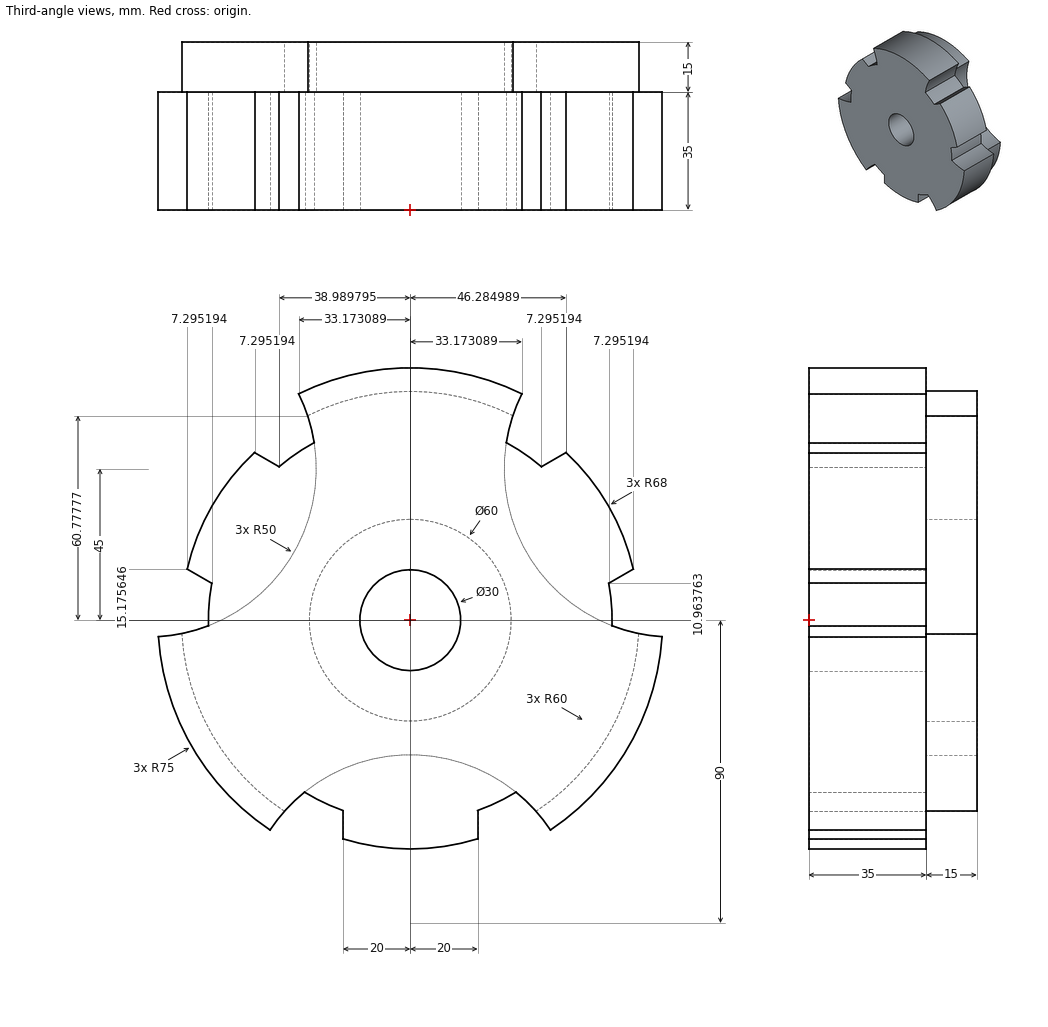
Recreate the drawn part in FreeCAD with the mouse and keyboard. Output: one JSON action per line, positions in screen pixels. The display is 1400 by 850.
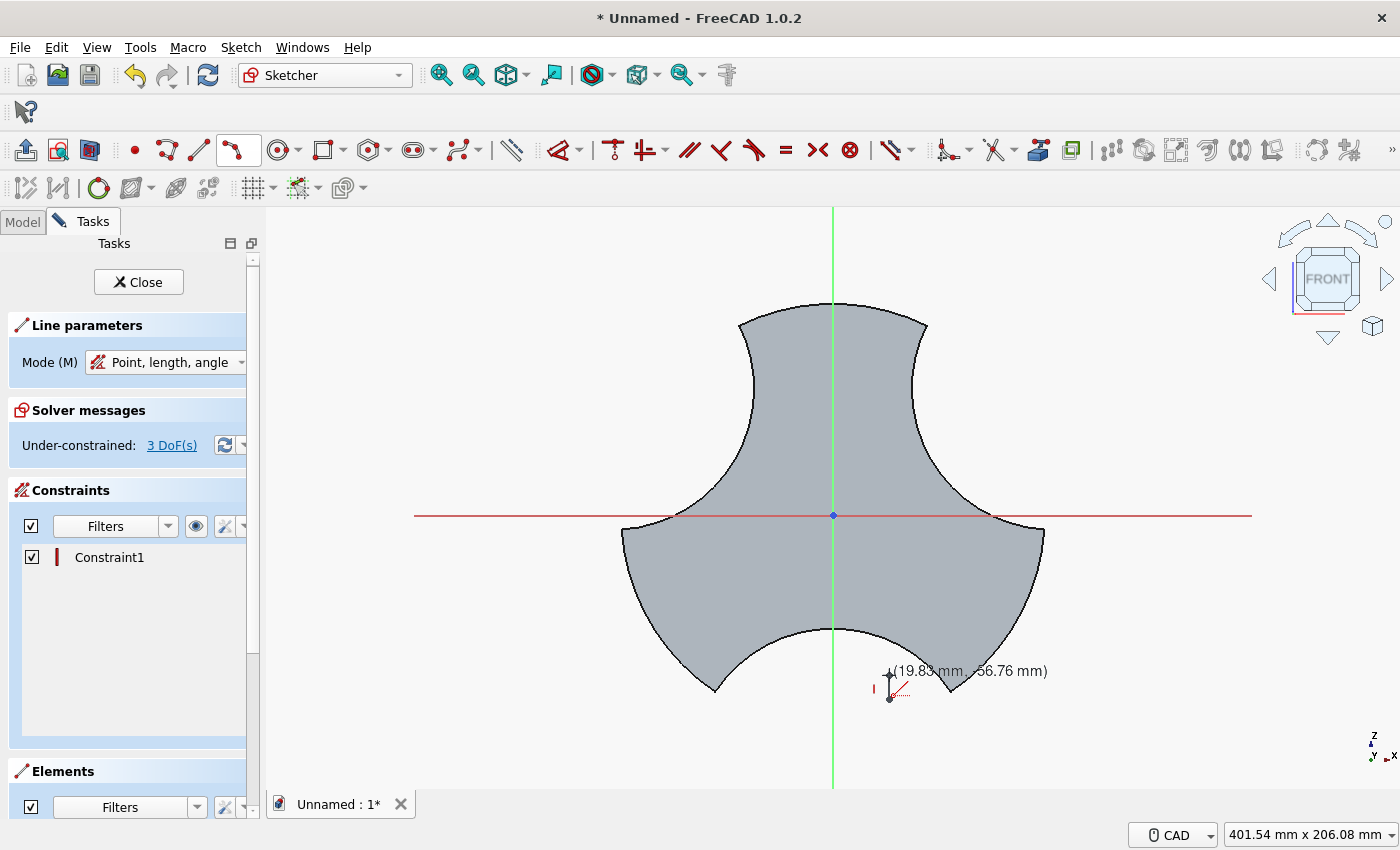
{"action": "left_click", "coordinate": [1000, 485]}
{"action": "left_click", "coordinate": [1020, 473]}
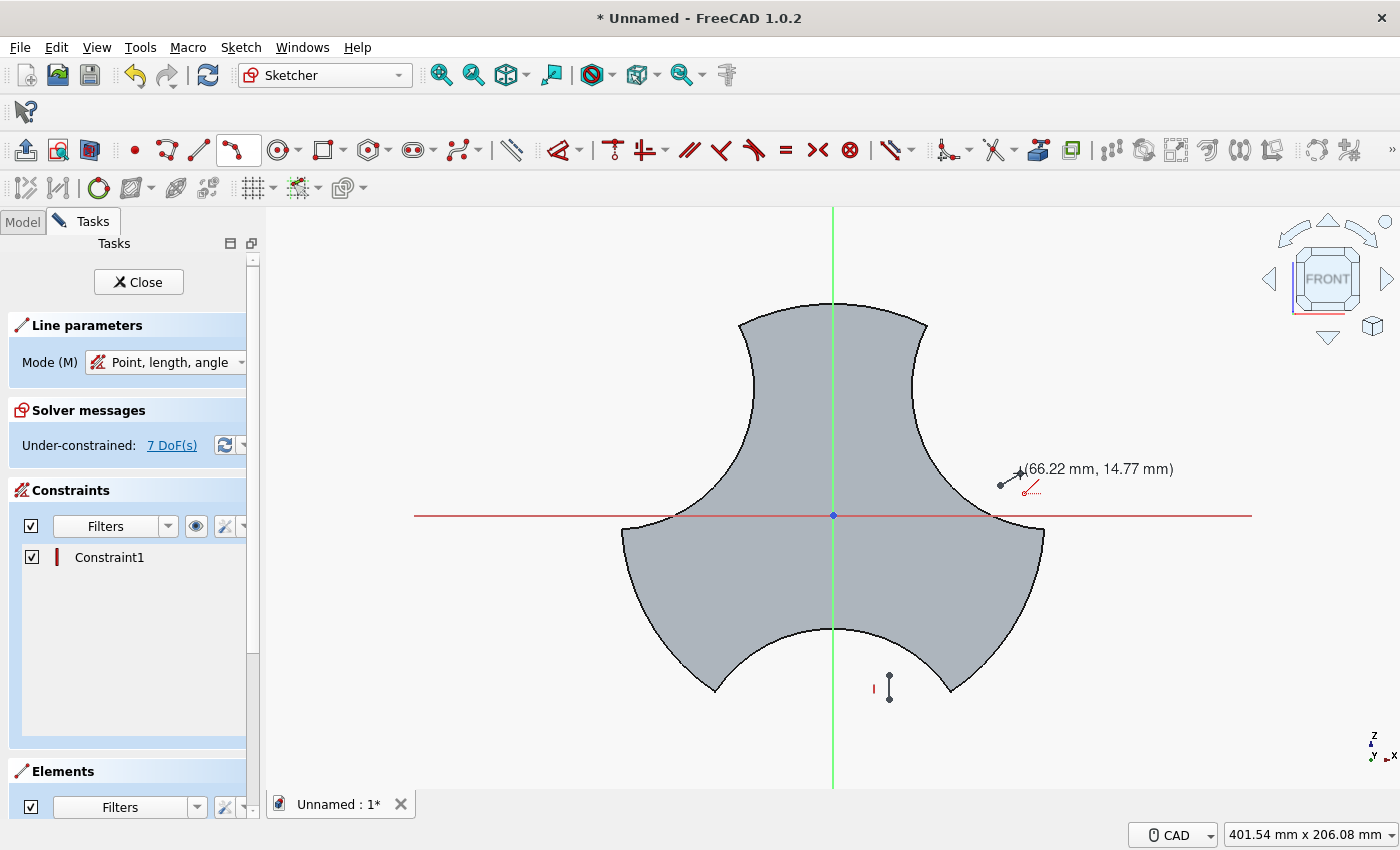
{"action": "left_click", "coordinate": [964, 375]}
{"action": "left_click", "coordinate": [943, 387]}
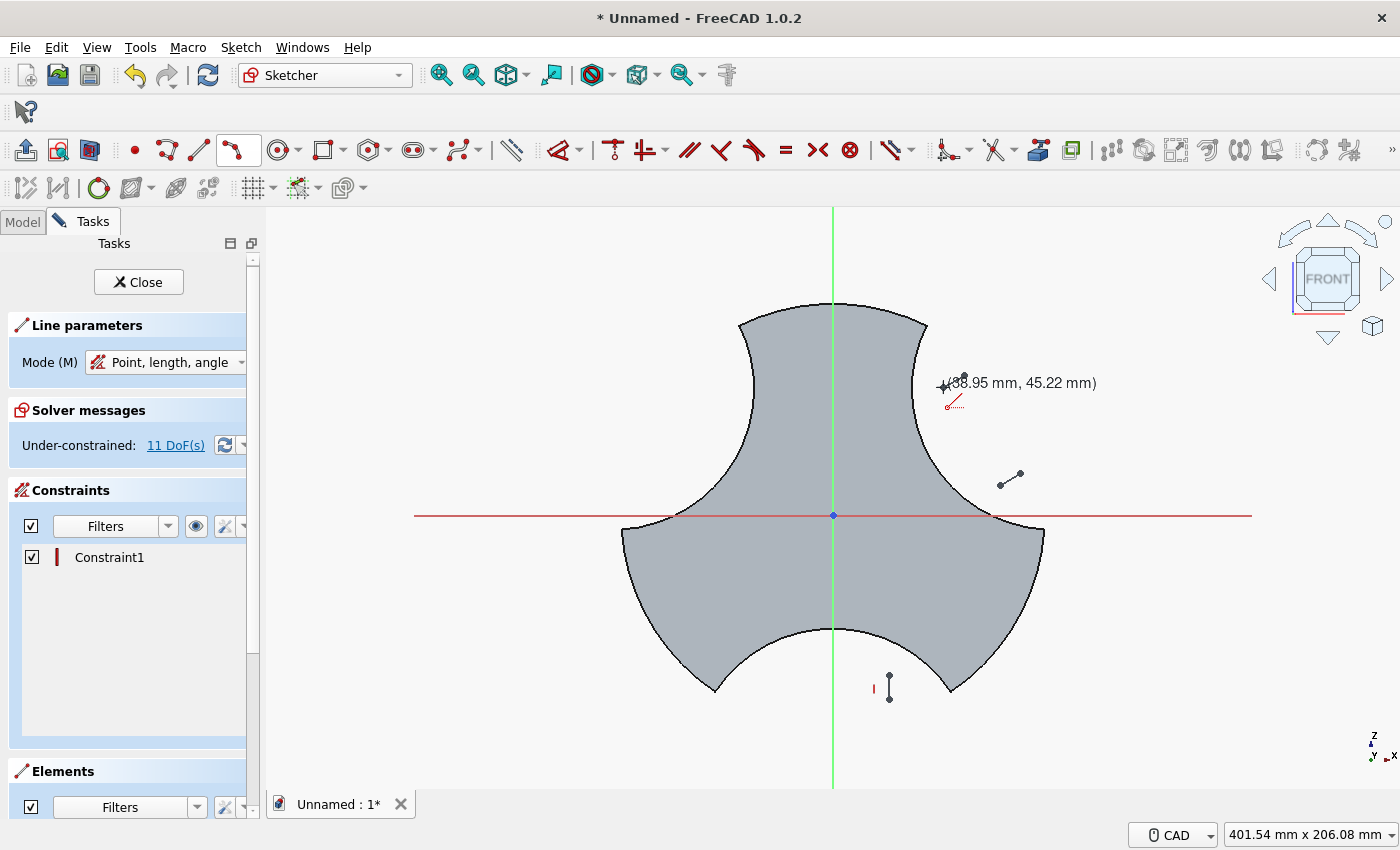
{"action": "left_click", "coordinate": [723, 387]}
{"action": "left_click", "coordinate": [702, 375]}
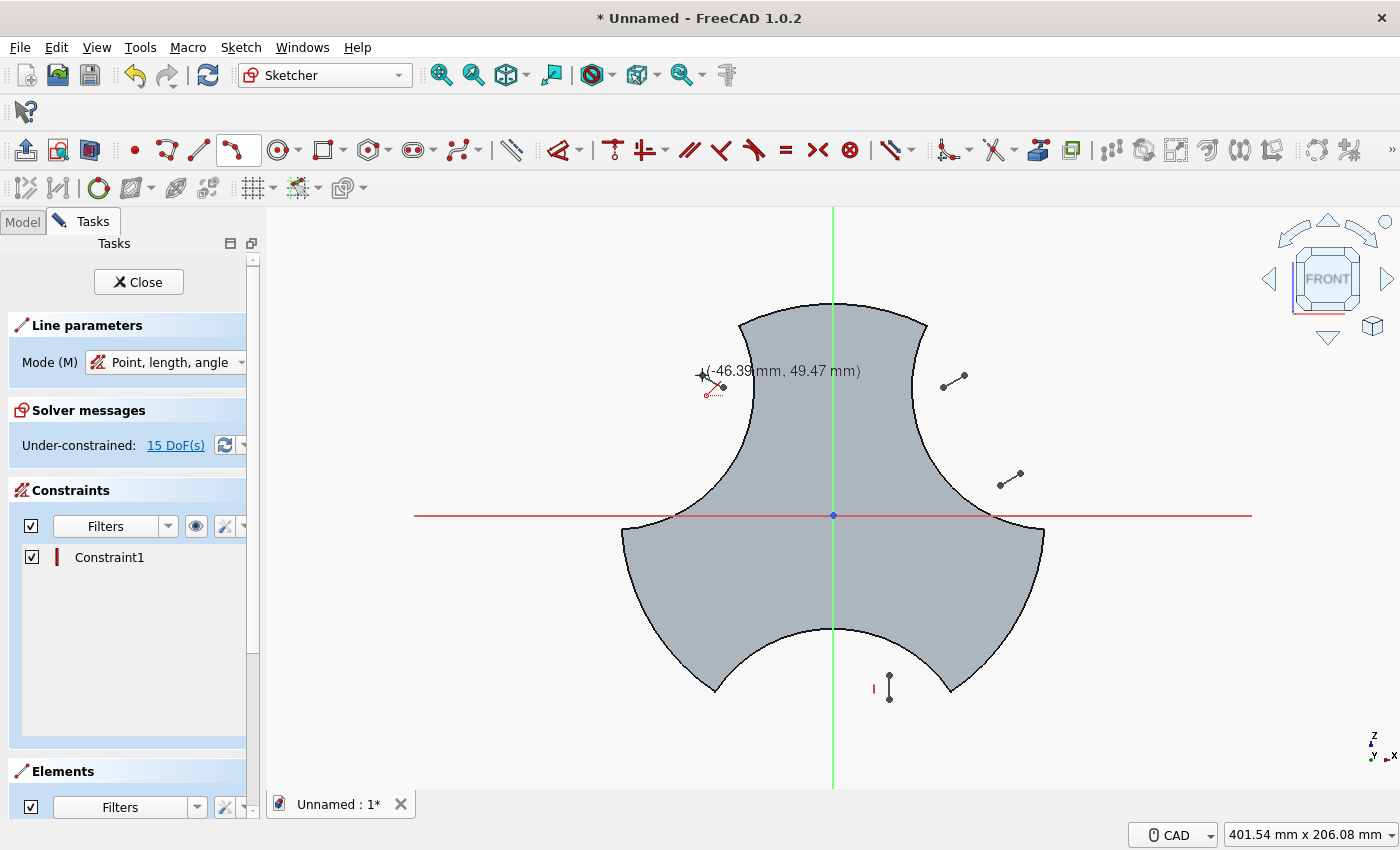
{"action": "left_click", "coordinate": [646, 473]}
{"action": "left_click", "coordinate": [666, 485]}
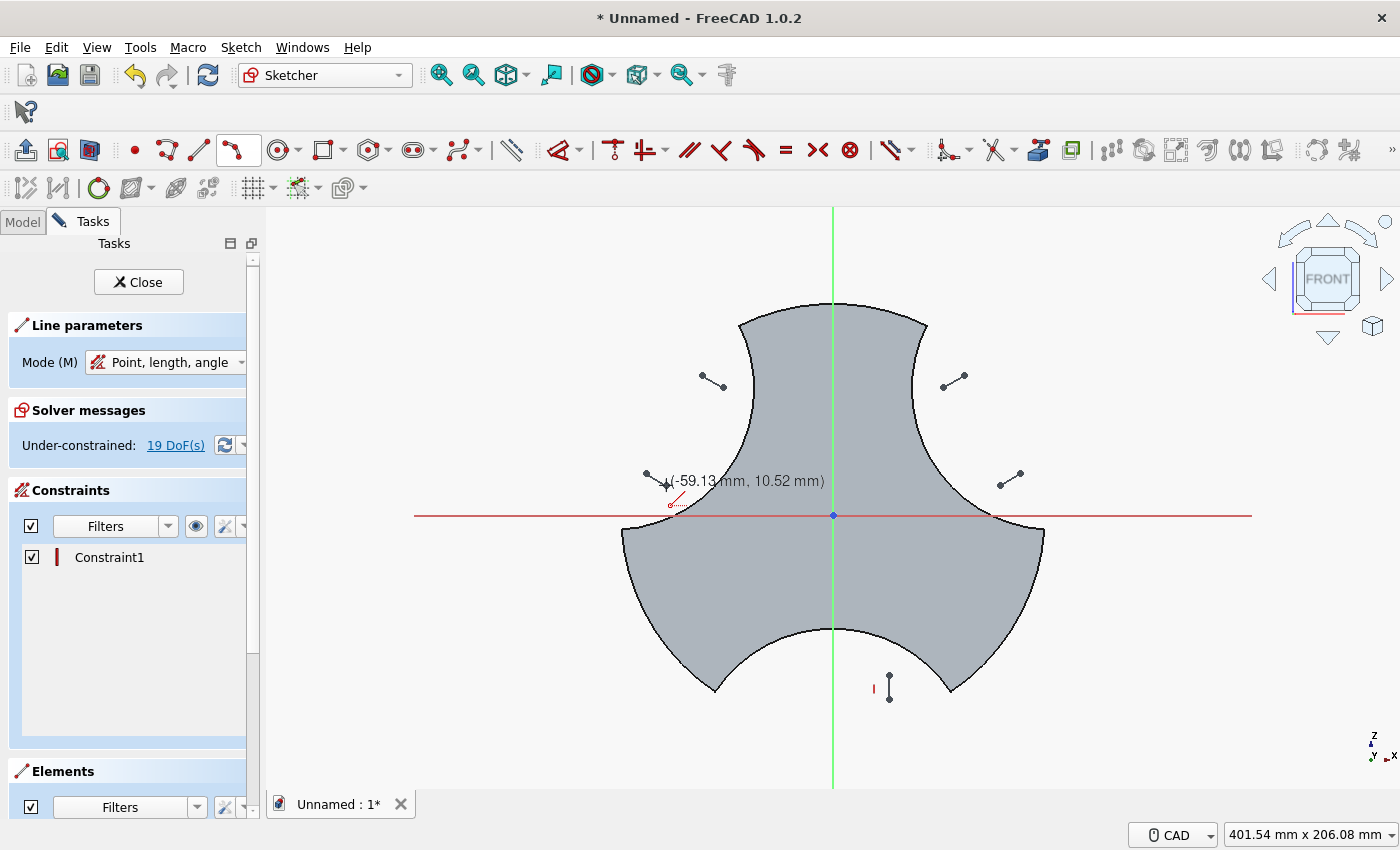
{"action": "left_click", "coordinate": [777, 675]}
{"action": "left_click", "coordinate": [777, 699]}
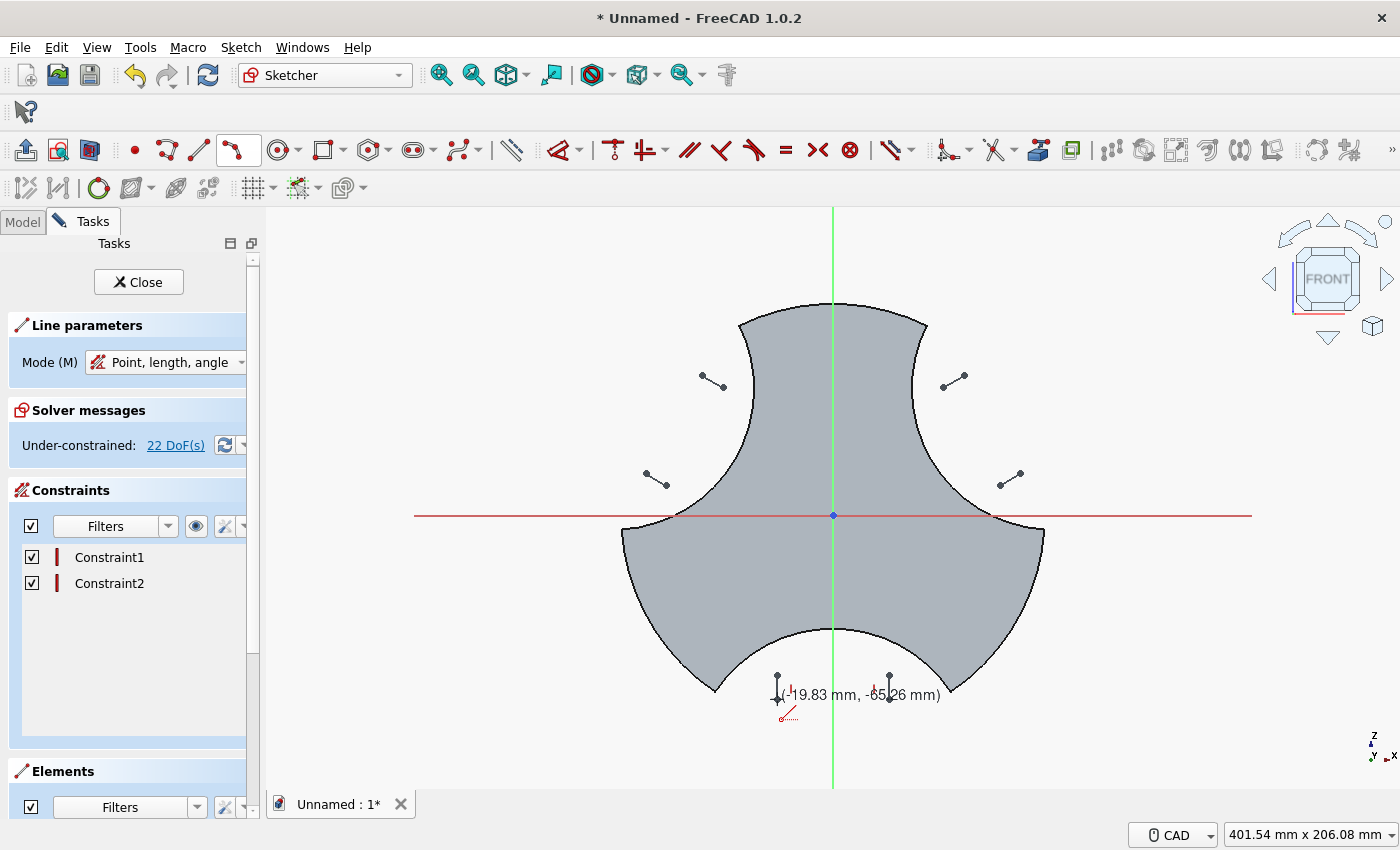
{"action": "left_click", "coordinate": [232, 150]}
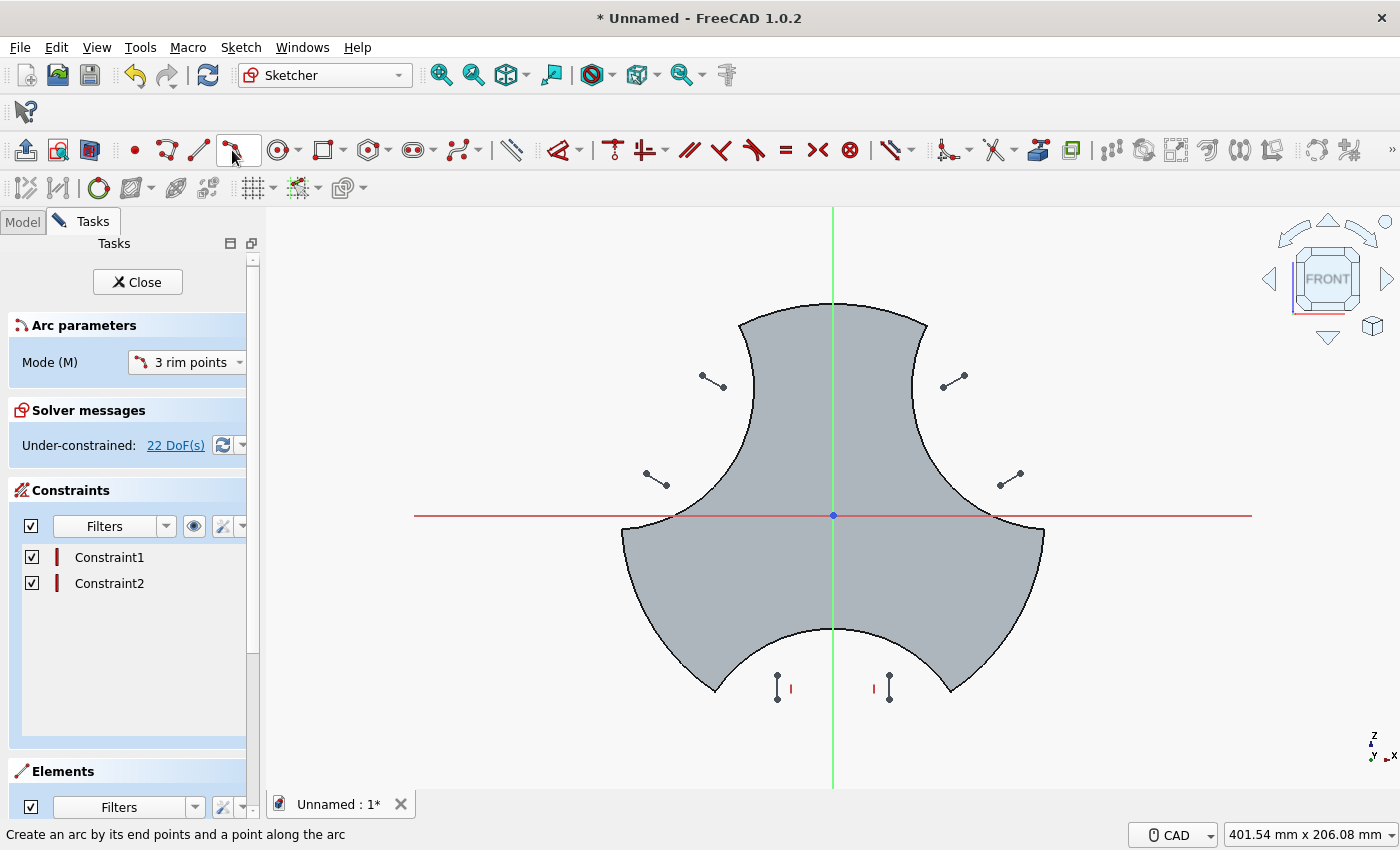
{"action": "scroll", "coordinate": [889, 675], "scroll_direction": "up", "scroll_amount": 2}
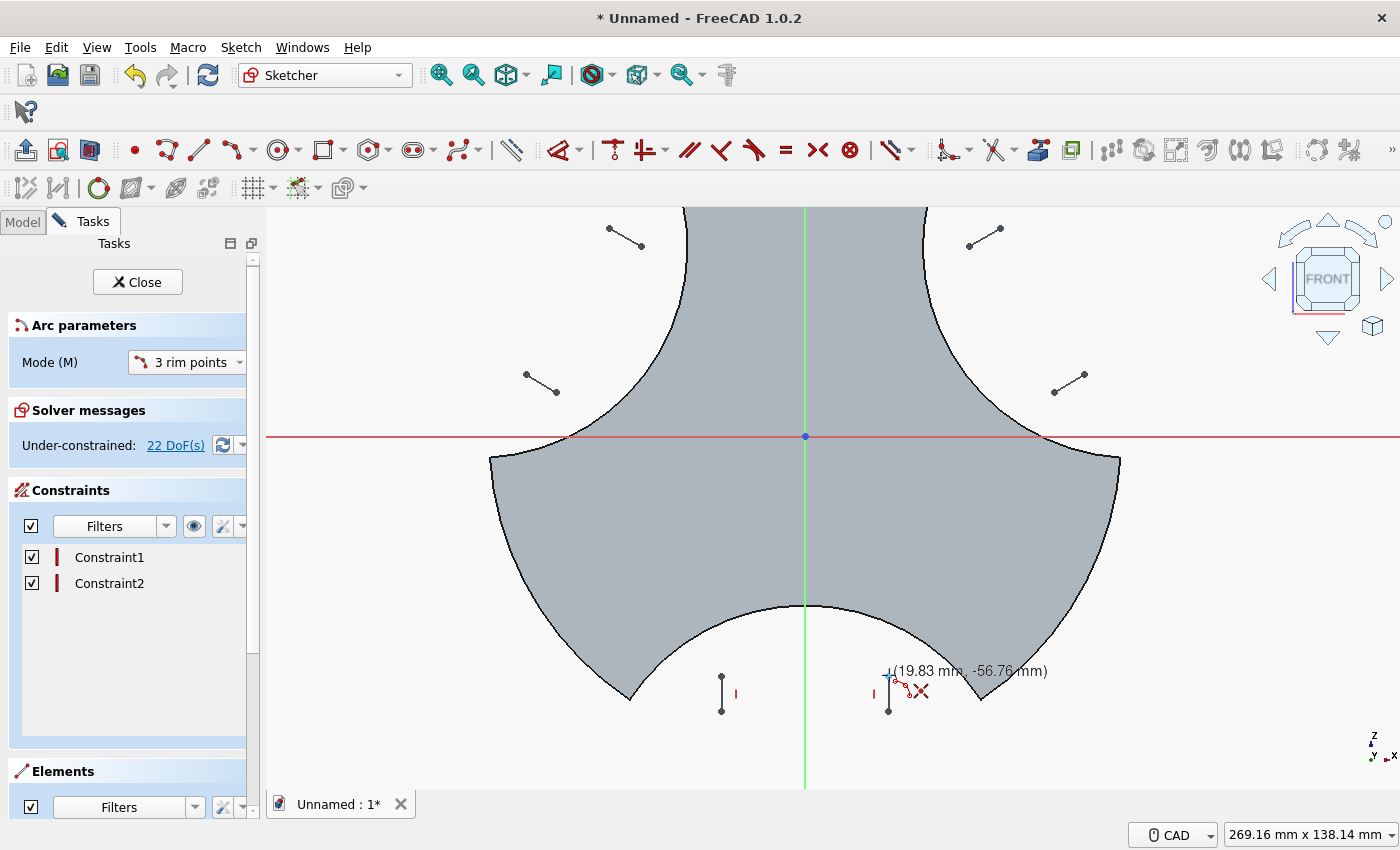
{"action": "left_click", "coordinate": [889, 676]}
{"action": "left_click", "coordinate": [1054, 393]}
{"action": "left_click", "coordinate": [1024, 563]}